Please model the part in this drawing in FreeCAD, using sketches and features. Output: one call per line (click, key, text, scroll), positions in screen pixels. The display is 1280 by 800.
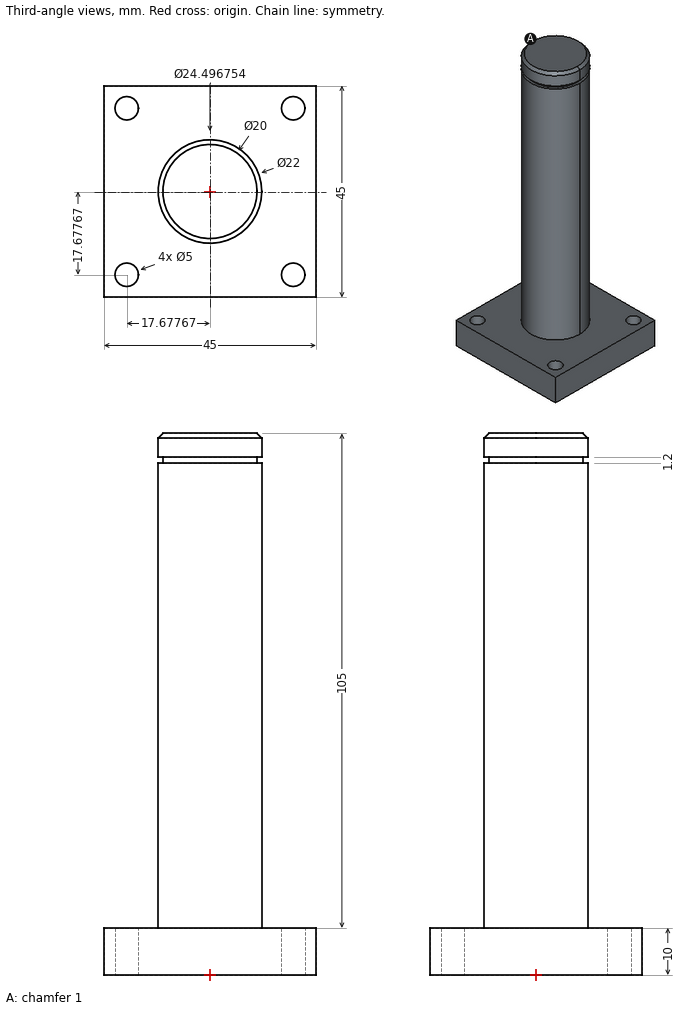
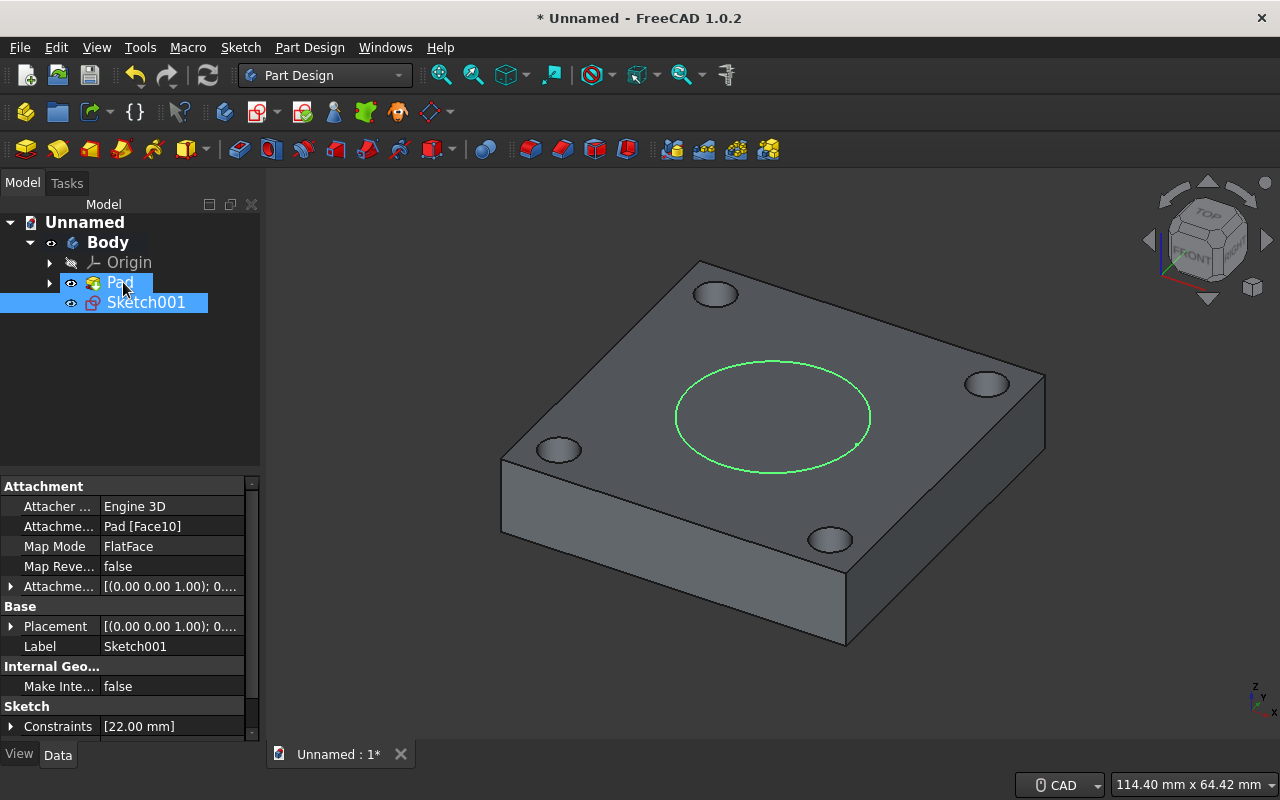
click(26, 150)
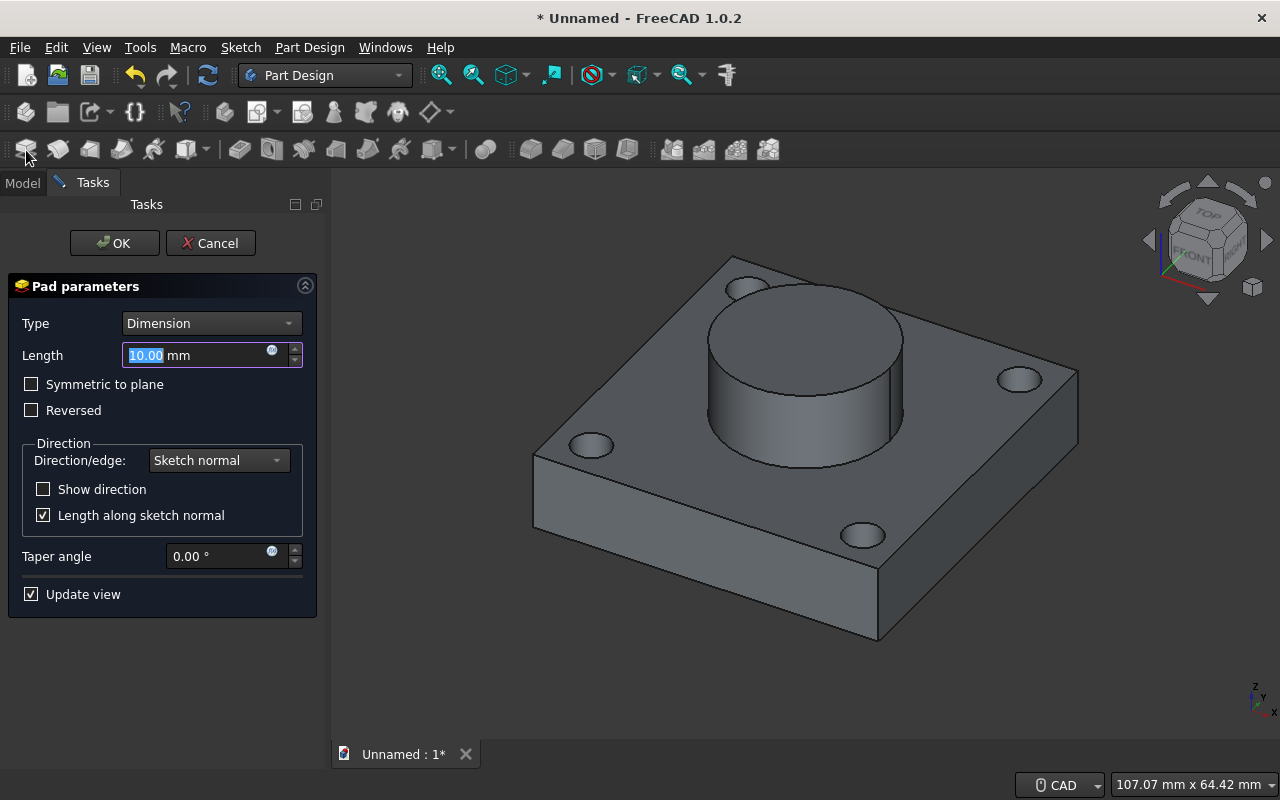
text(105)
key(Tab)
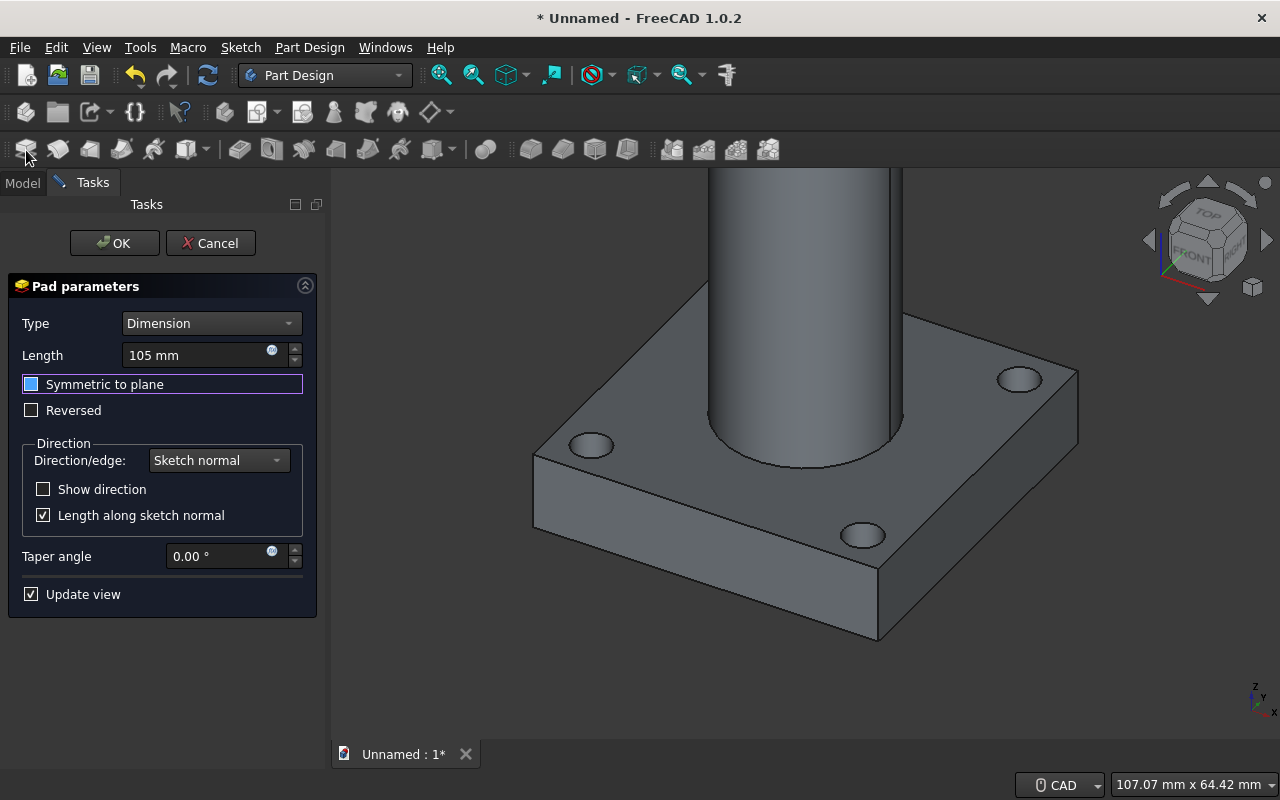
click(115, 243)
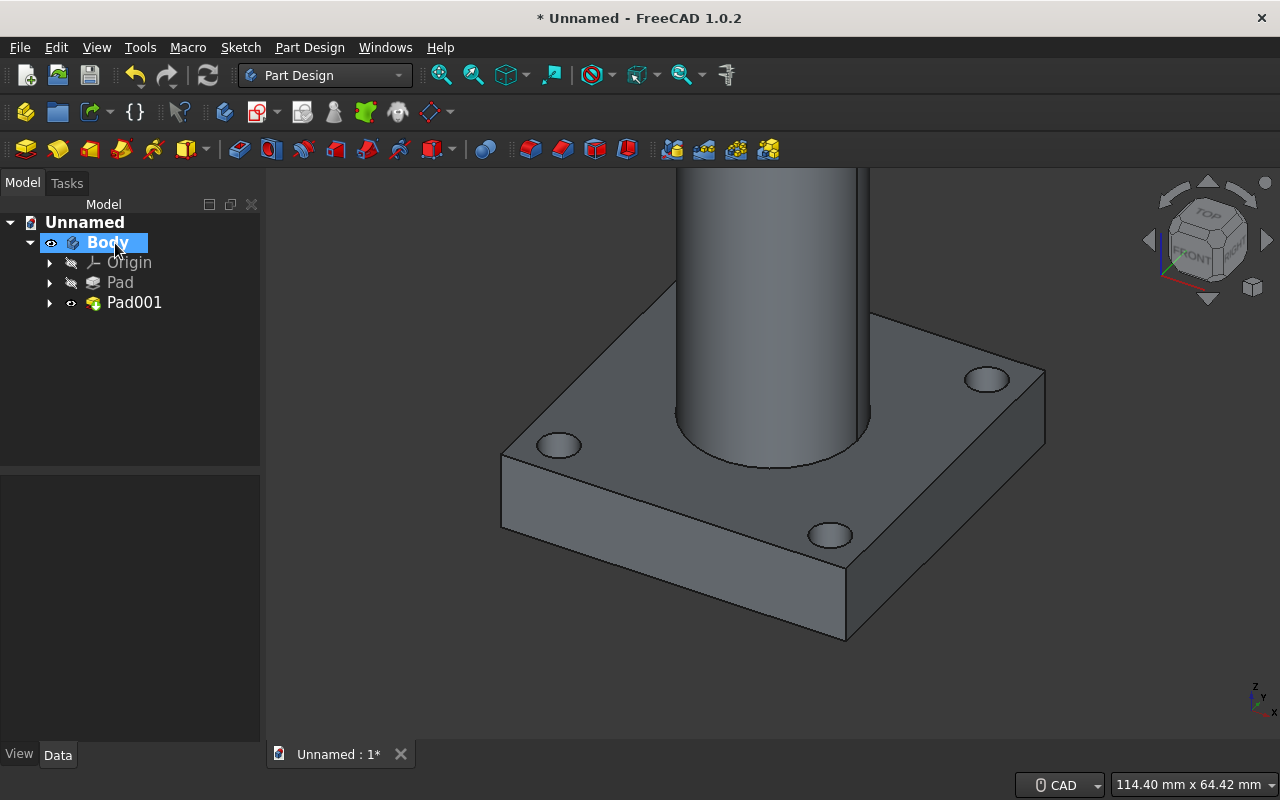
click(442, 76)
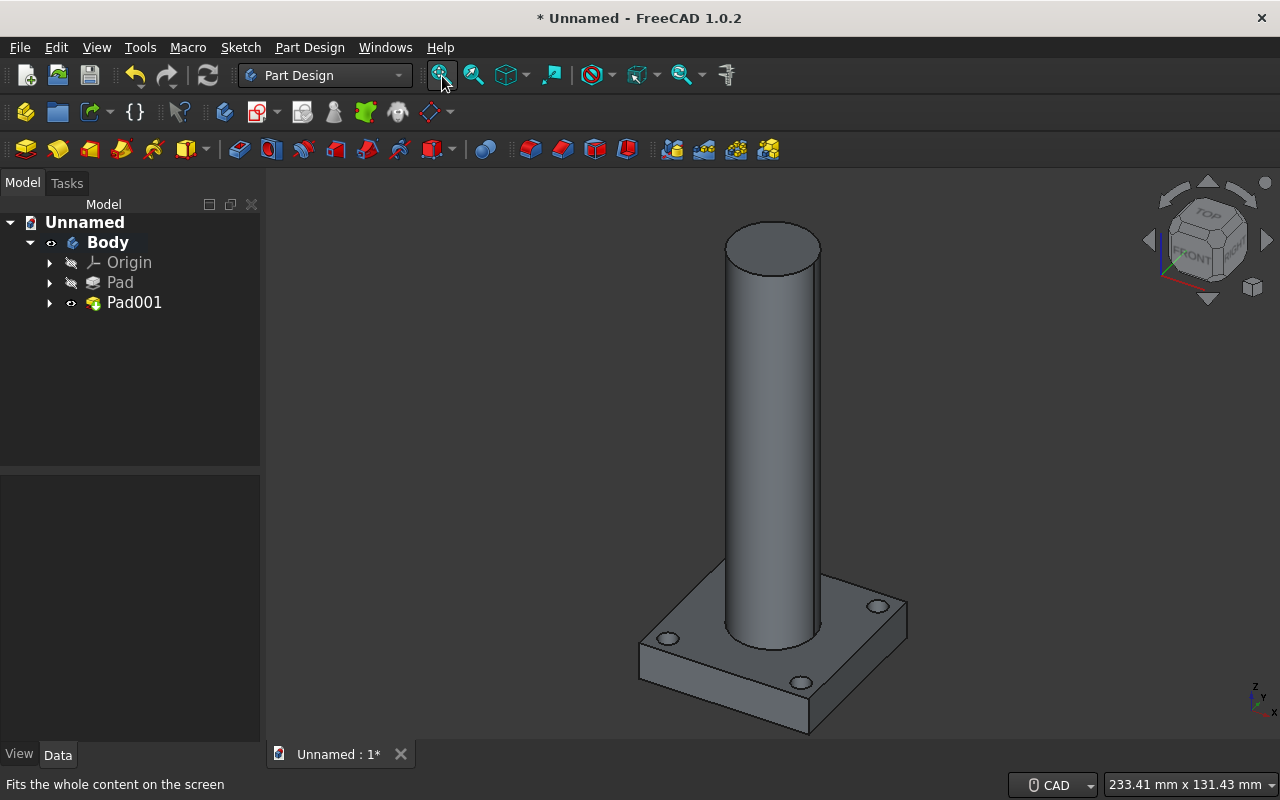
click(725, 251)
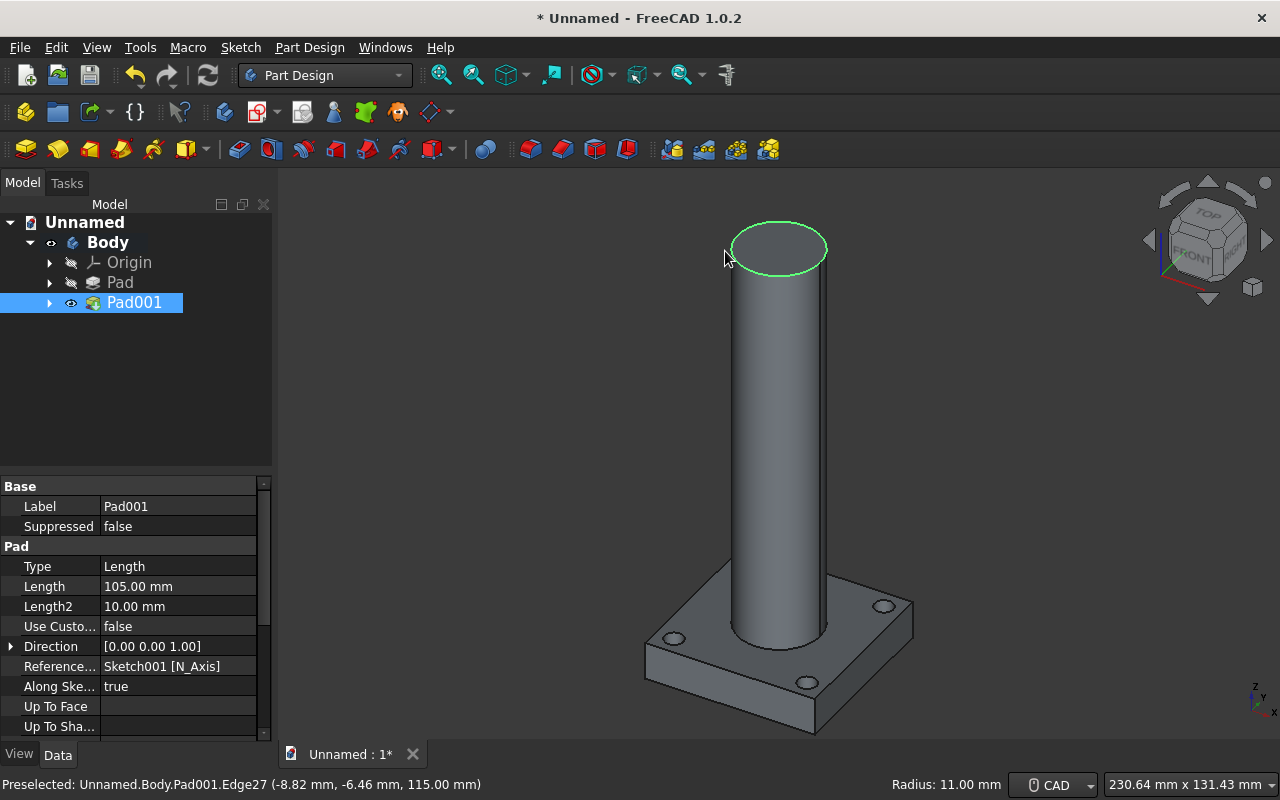
click(564, 150)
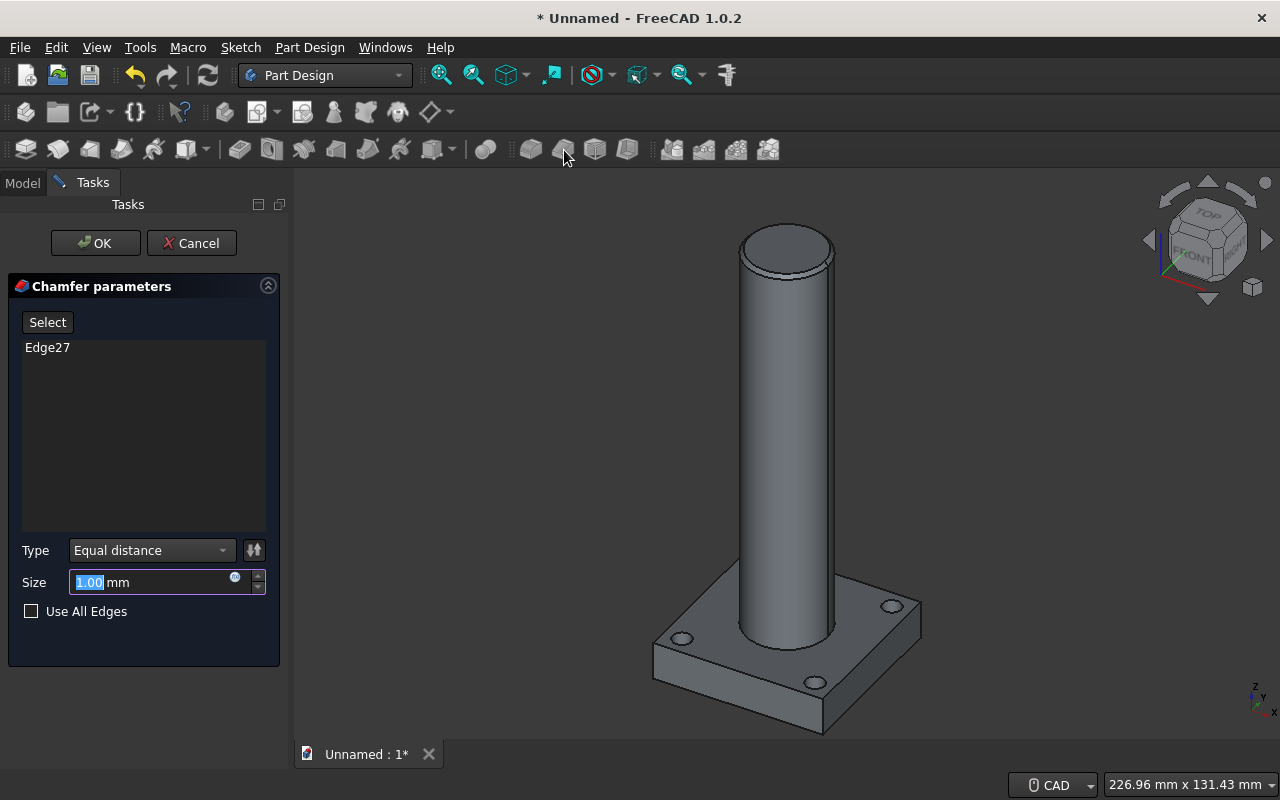
text(1)
key(Tab)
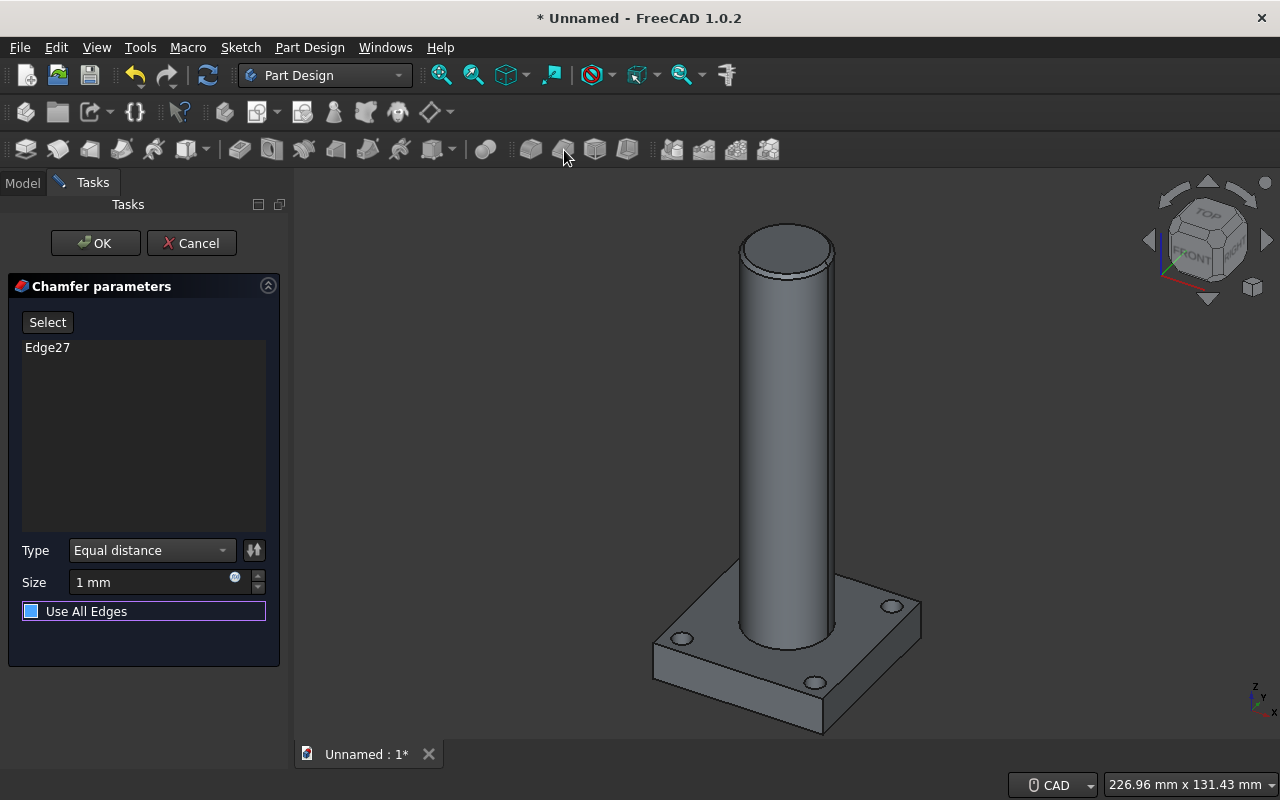
click(96, 243)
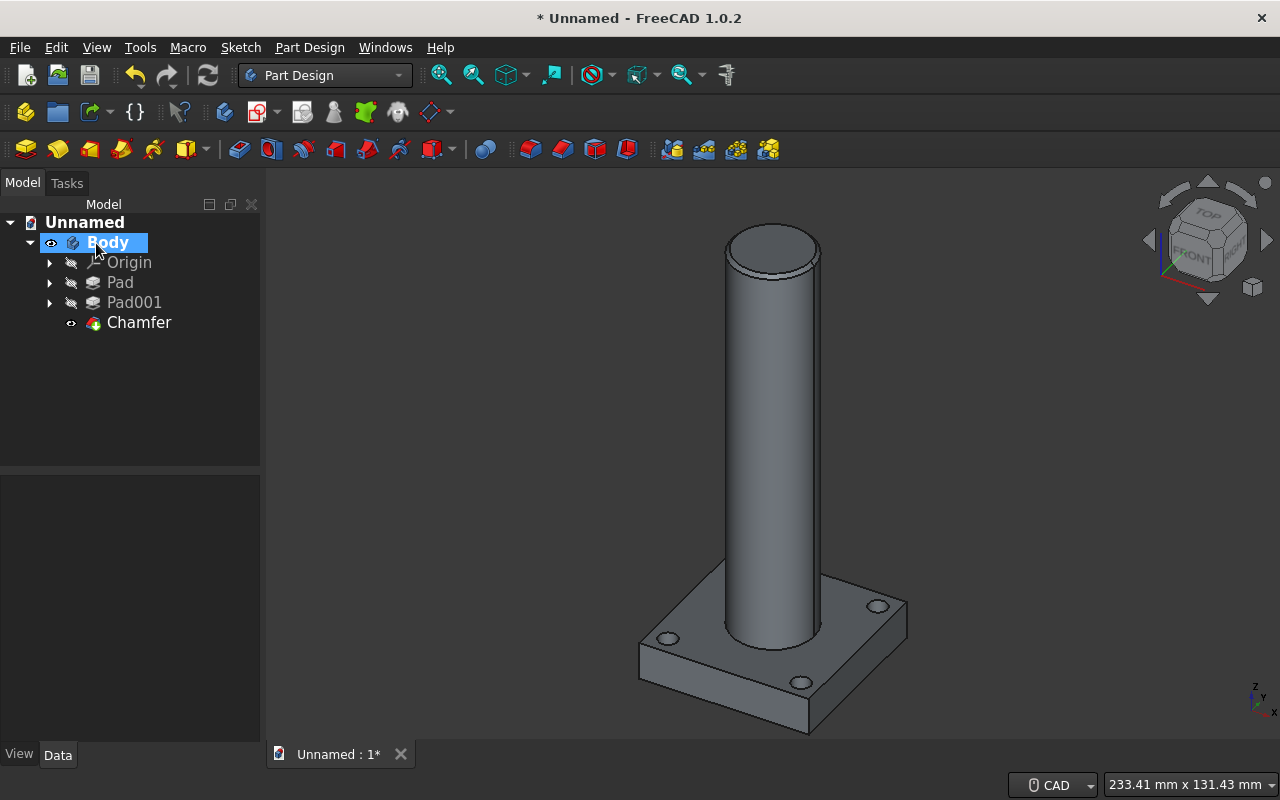
click(50, 263)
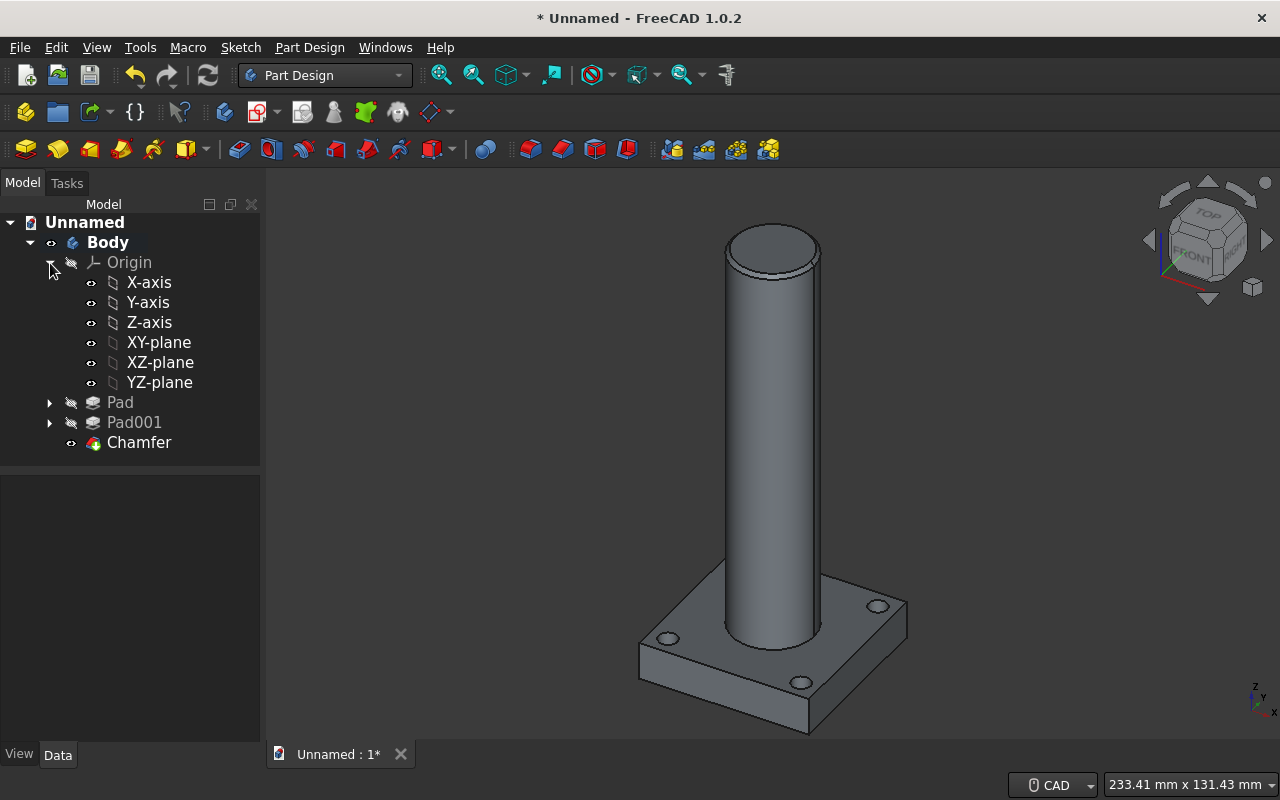
click(136, 343)